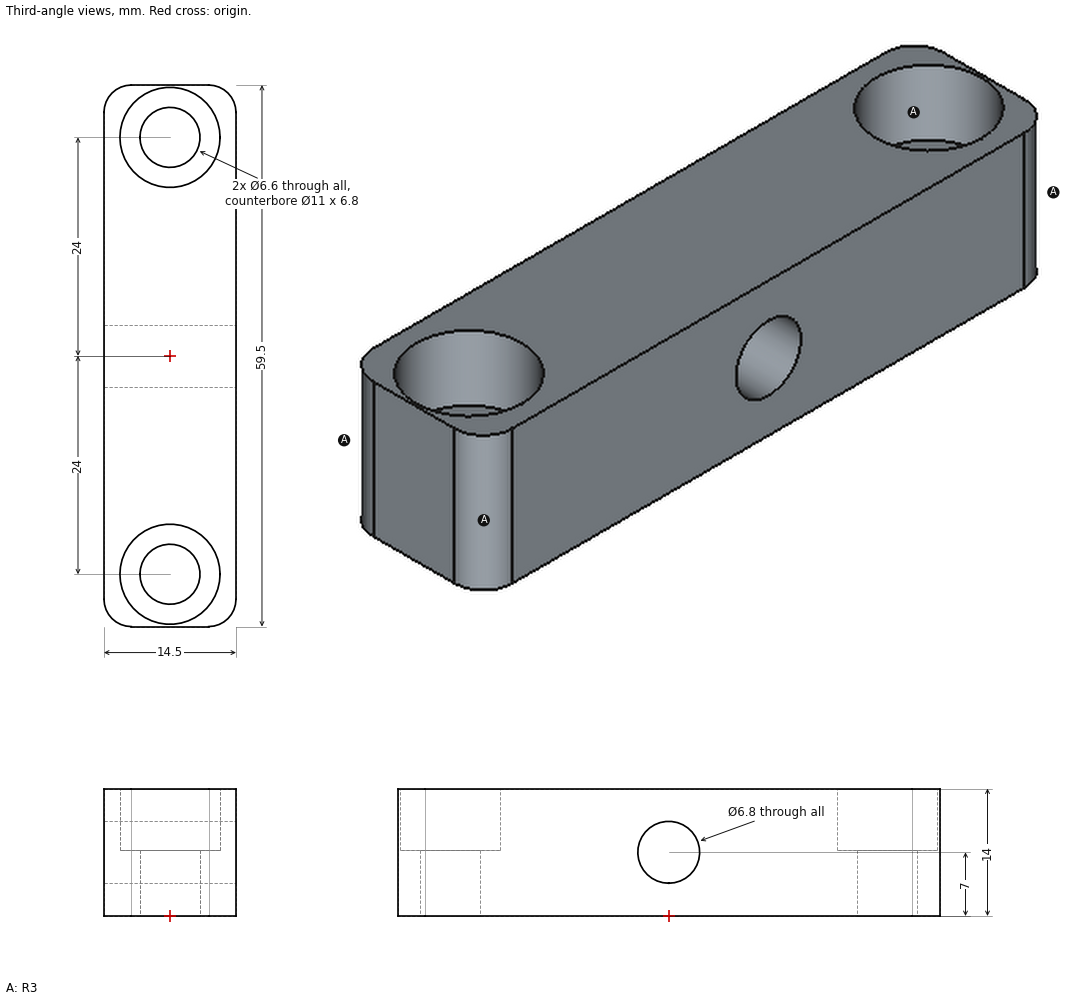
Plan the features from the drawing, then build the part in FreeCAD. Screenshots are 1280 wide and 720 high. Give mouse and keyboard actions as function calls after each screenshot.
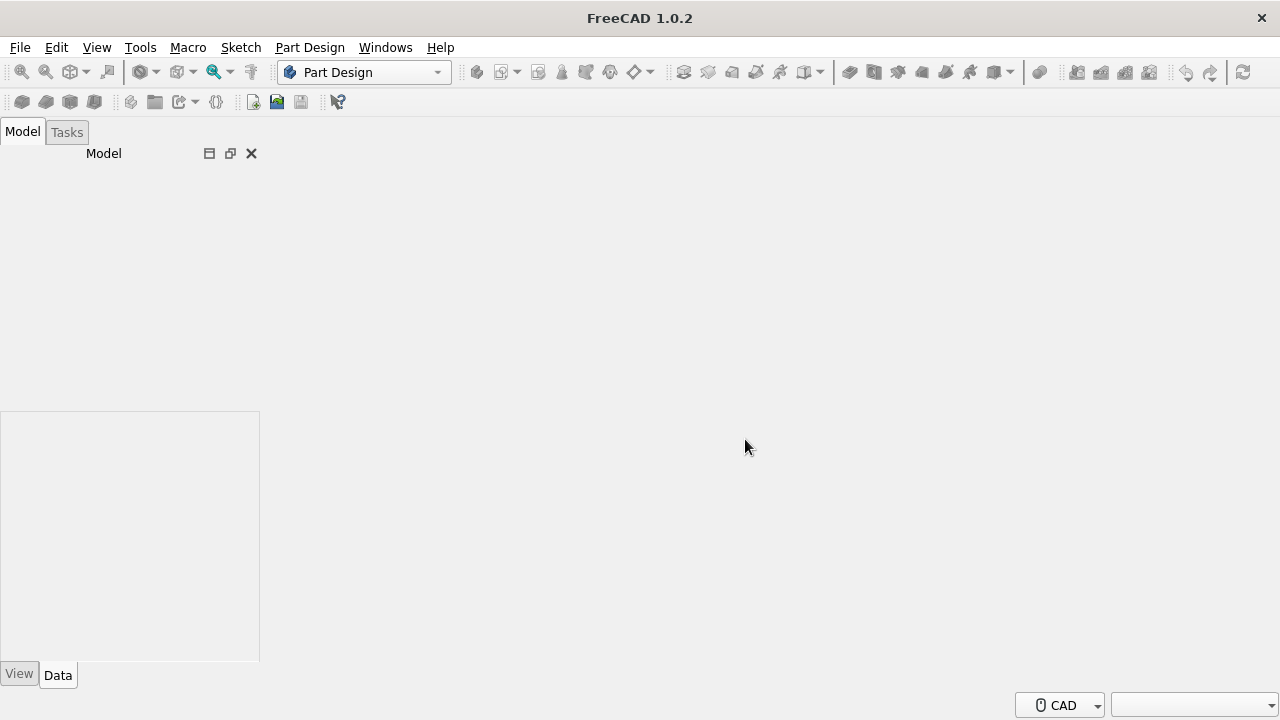
key(ctrl+n)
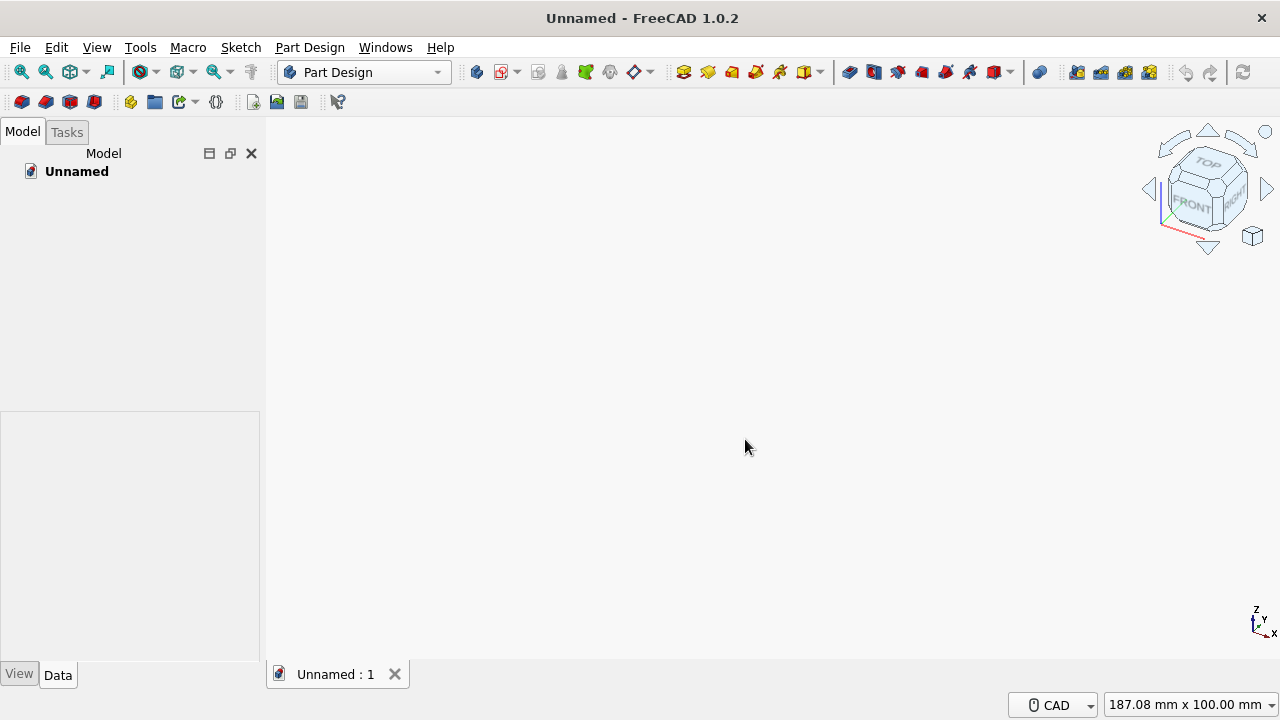
click(502, 72)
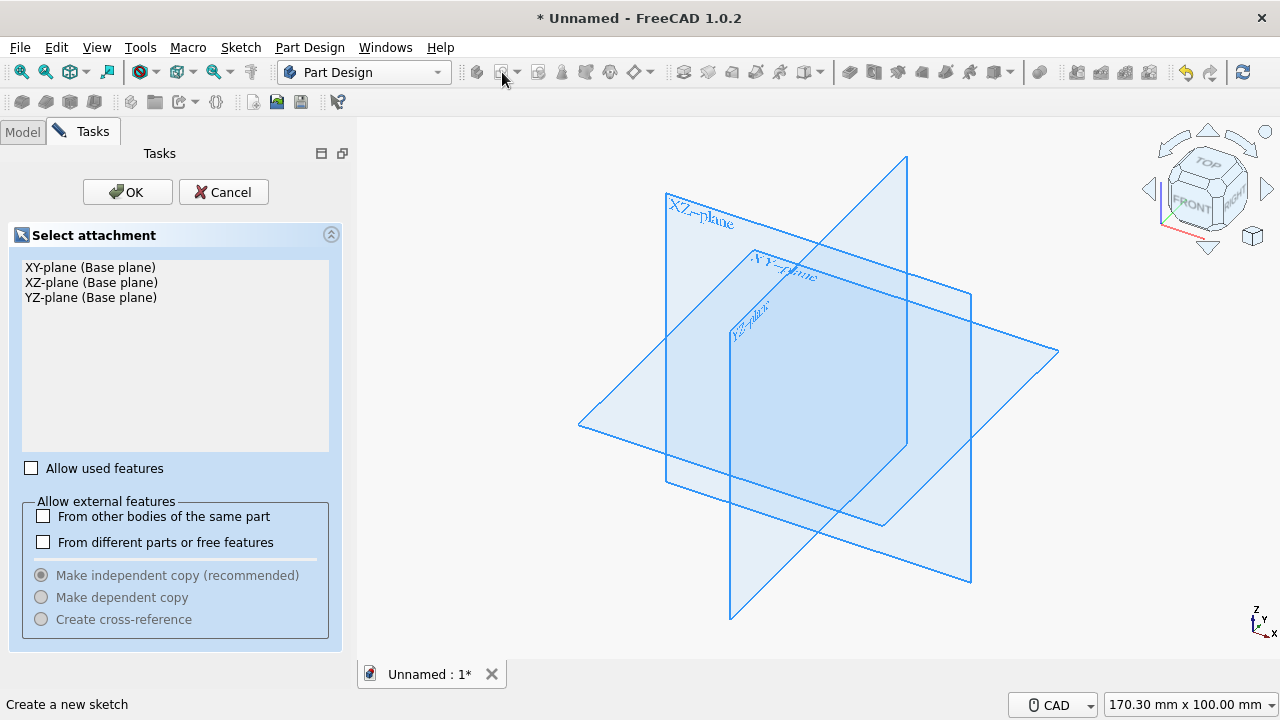
click(82, 268)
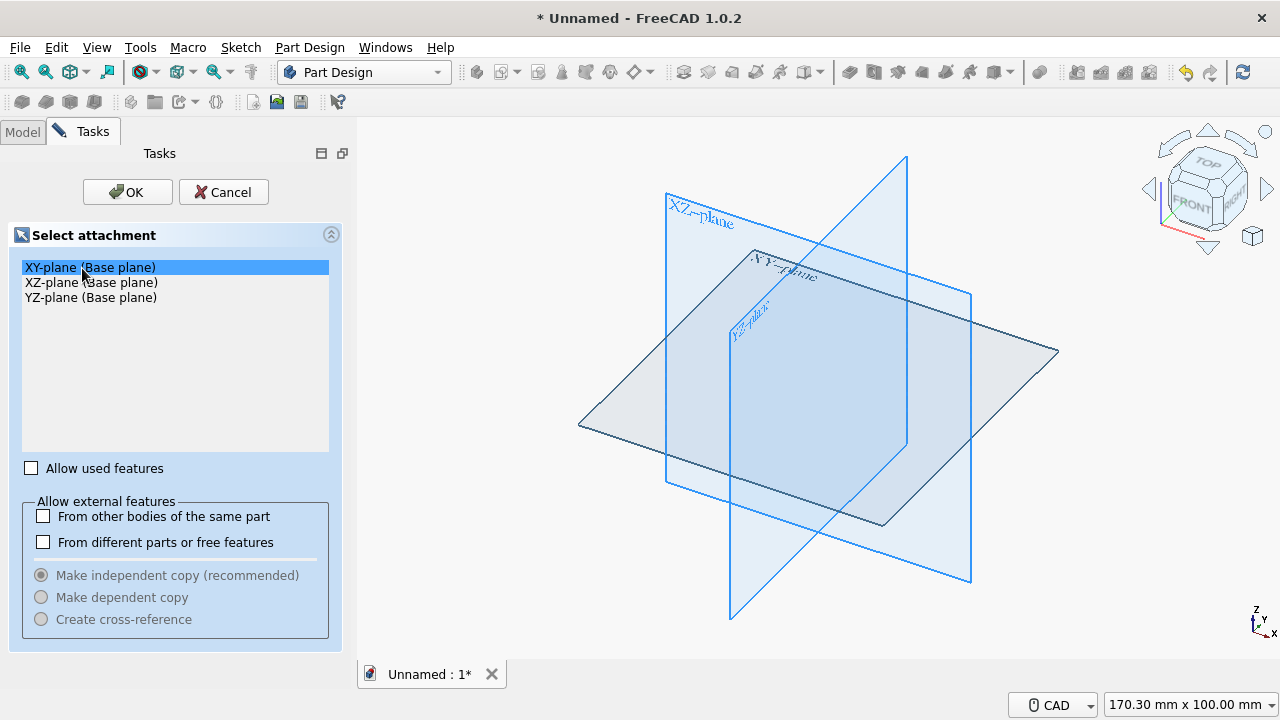
click(128, 192)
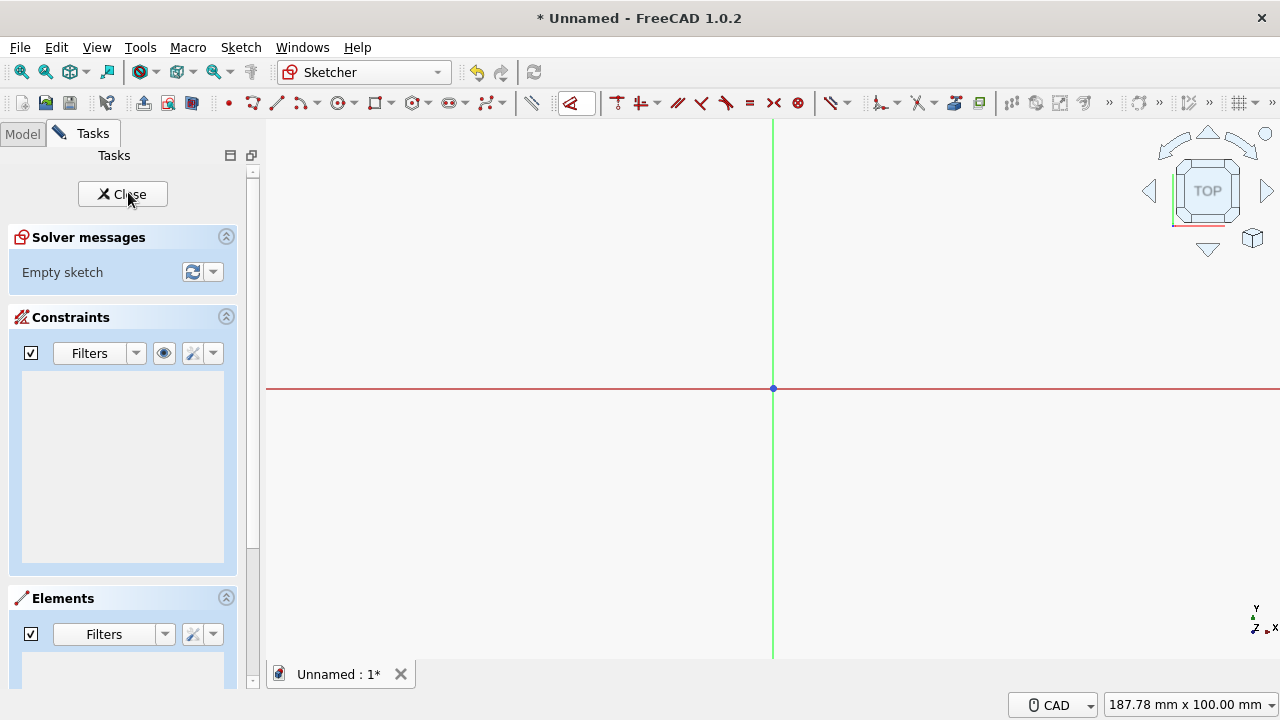
key(g)
key(v)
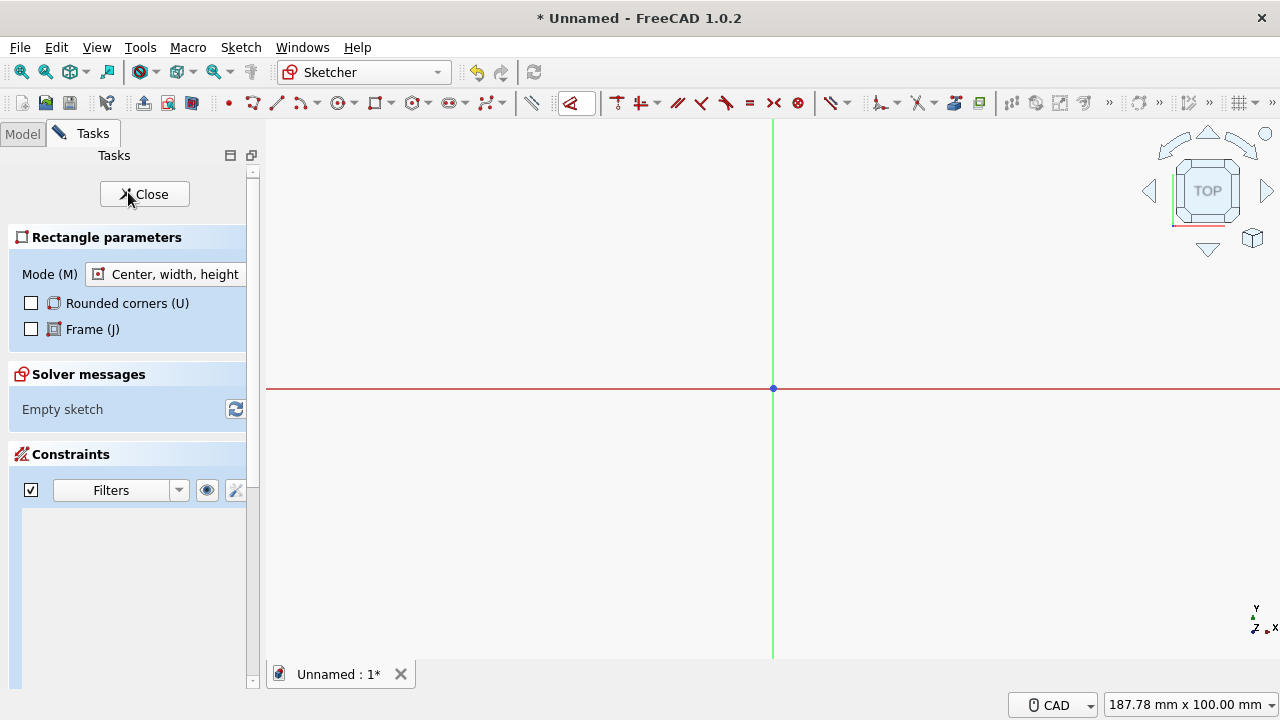
click(773, 389)
move(812, 228)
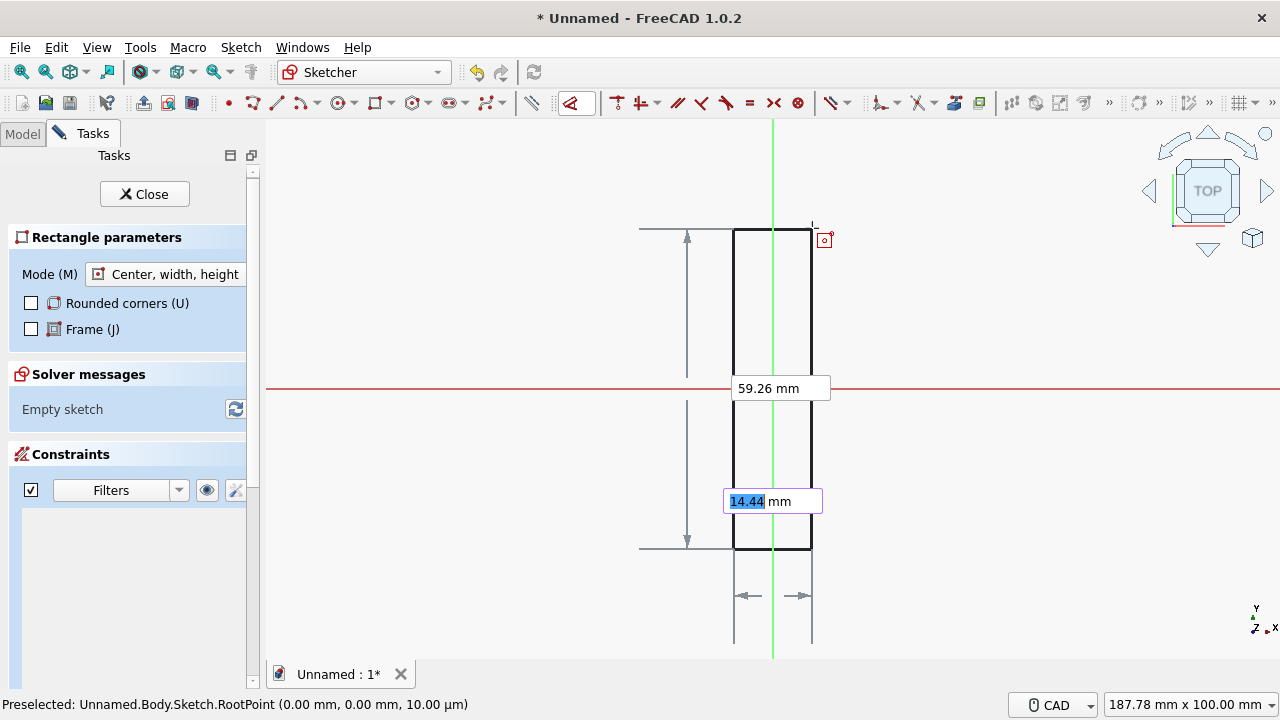
text(14.5)
key(Tab)
text(59.5)
key(Return)
key(Escape)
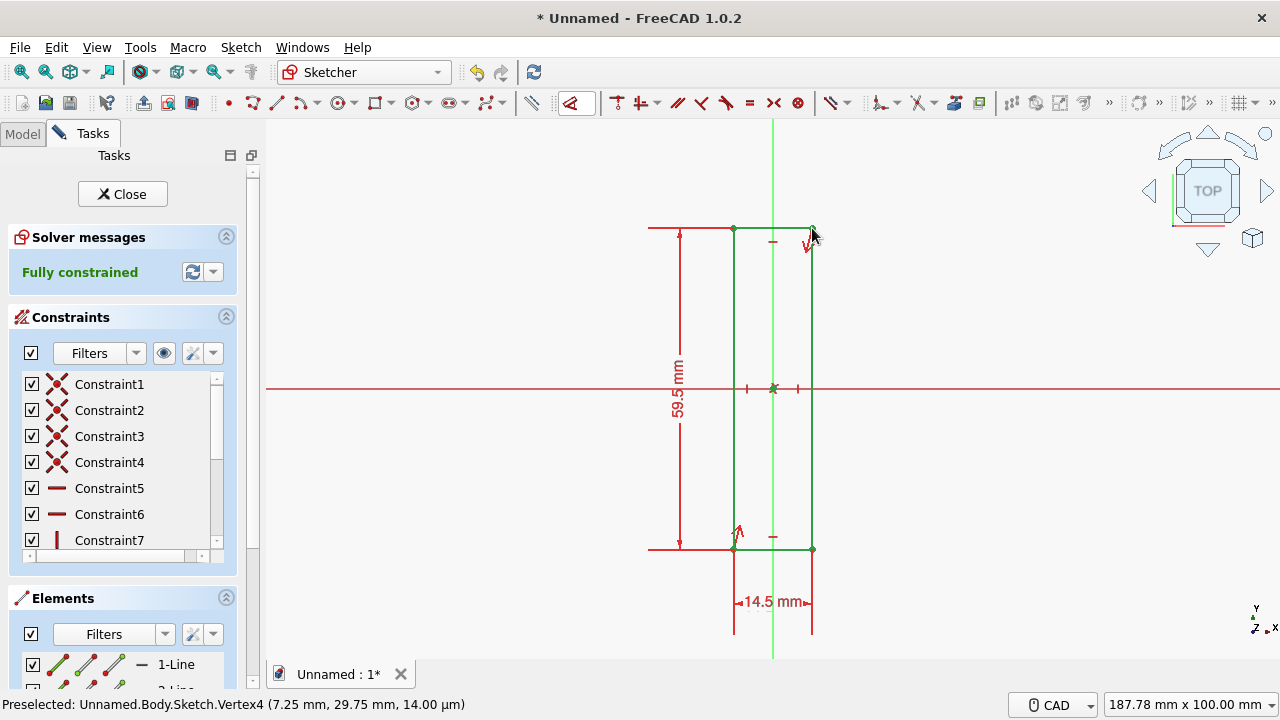
click(123, 194)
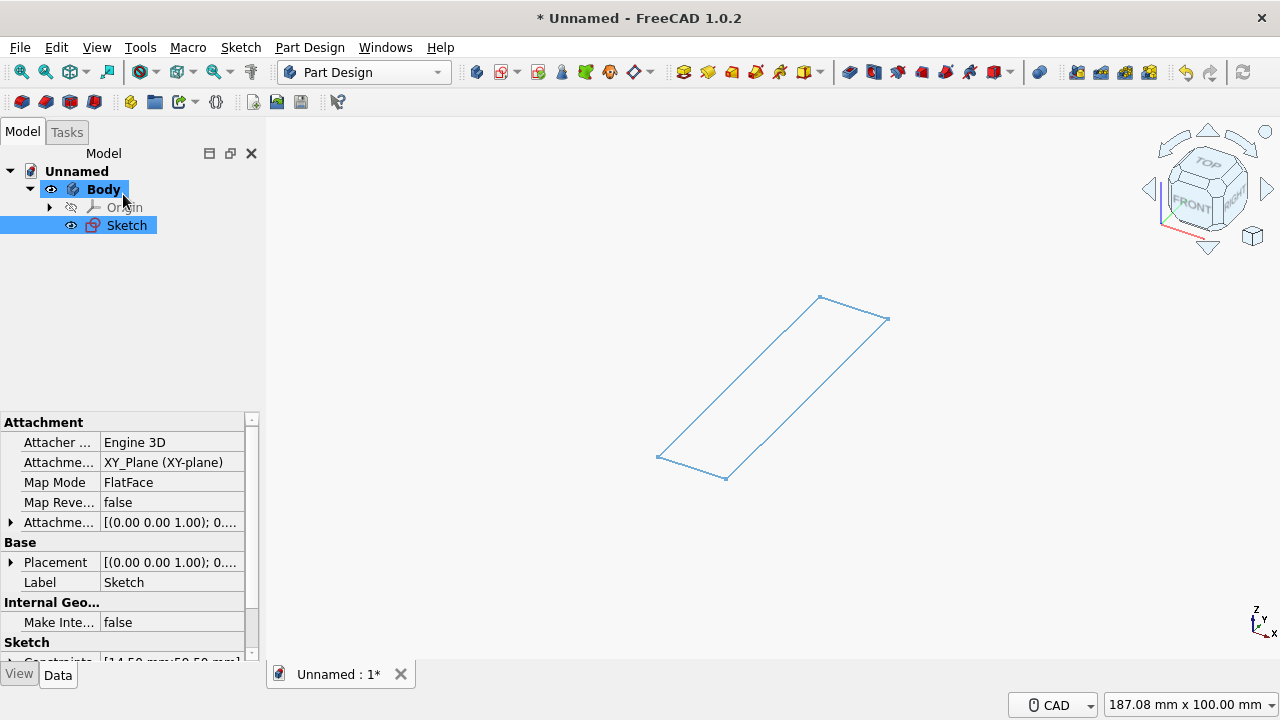
click(684, 72)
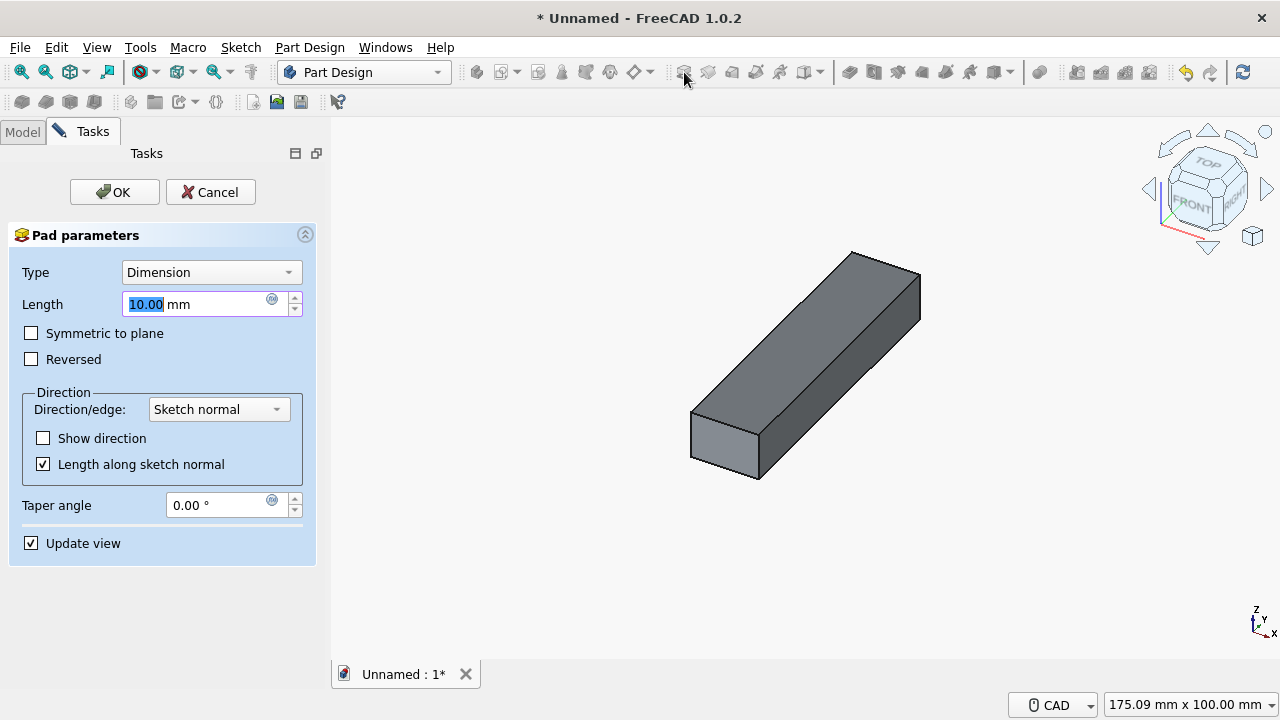
text(14)
key(Tab)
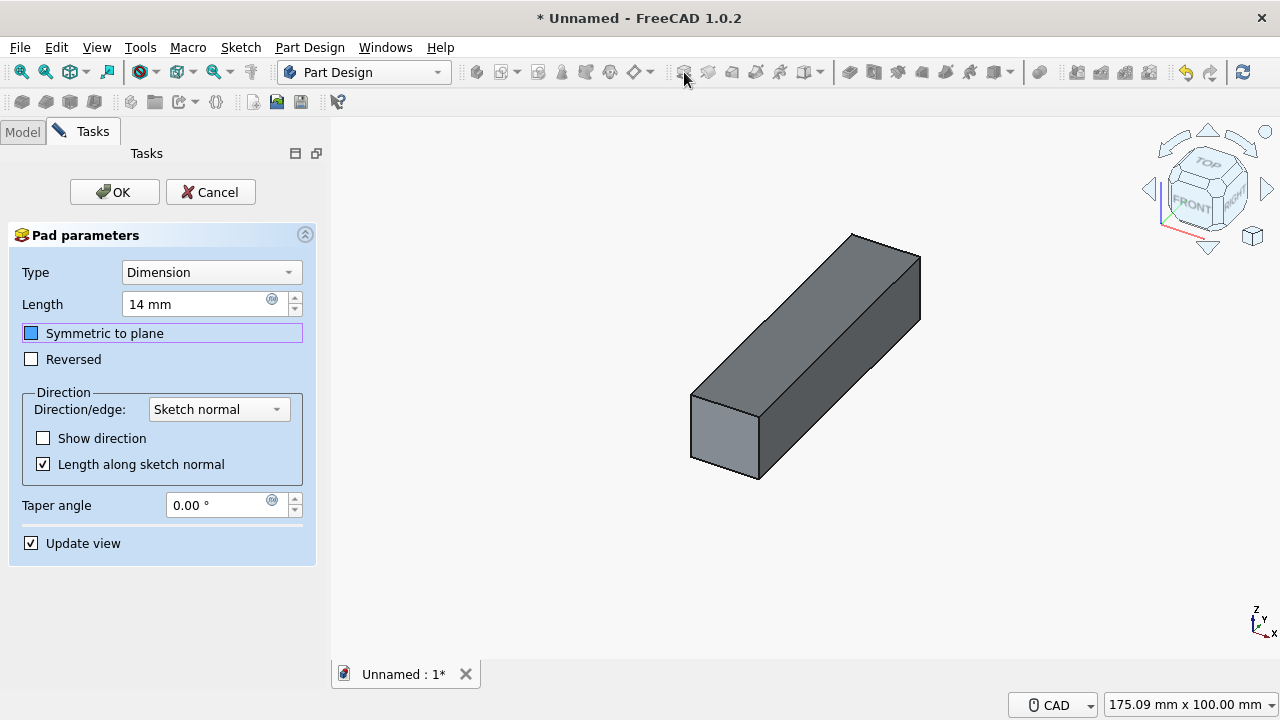
click(115, 192)